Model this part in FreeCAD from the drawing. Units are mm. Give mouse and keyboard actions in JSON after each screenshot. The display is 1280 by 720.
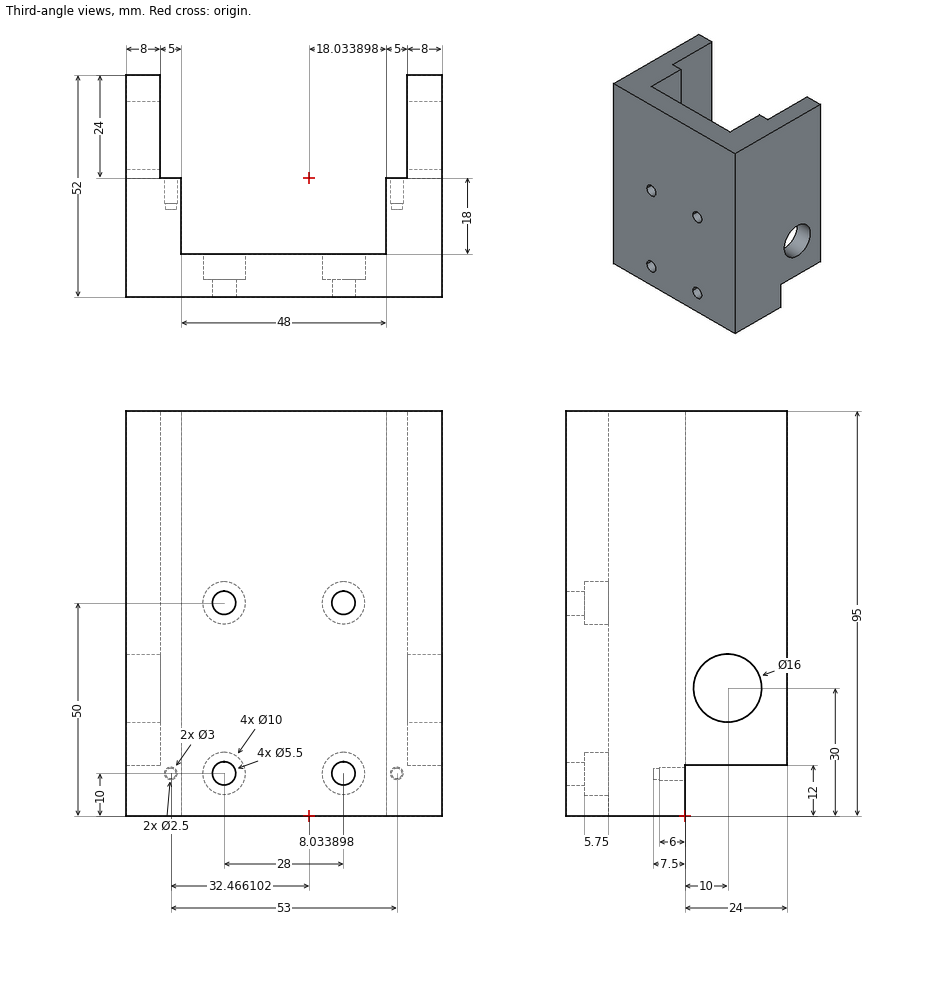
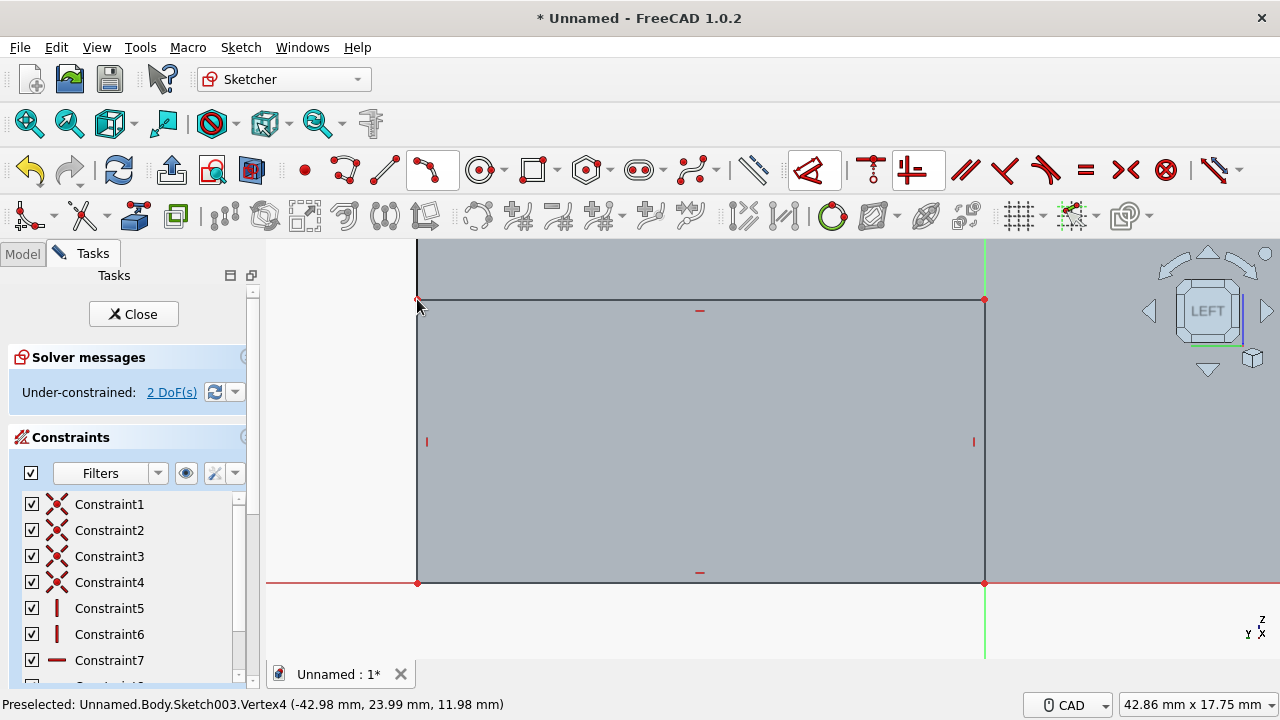
{"action": "left_click", "coordinate": [985, 498]}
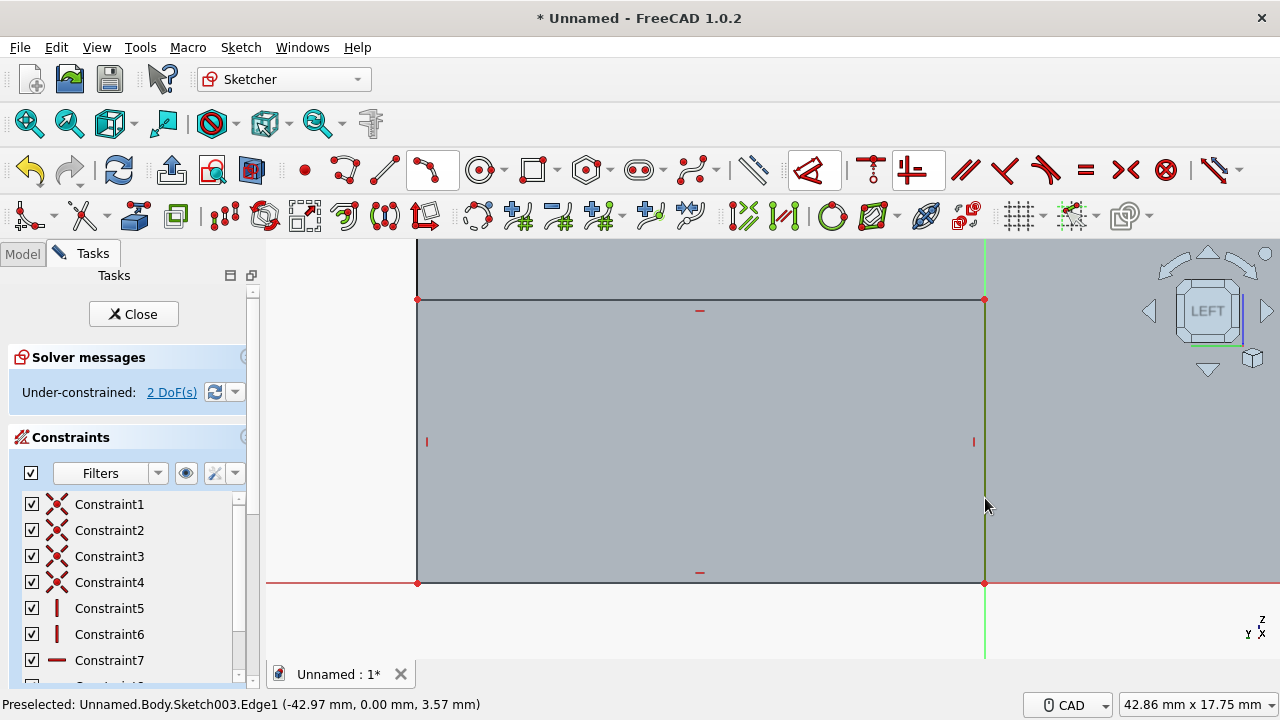
{"action": "key", "text": "i"}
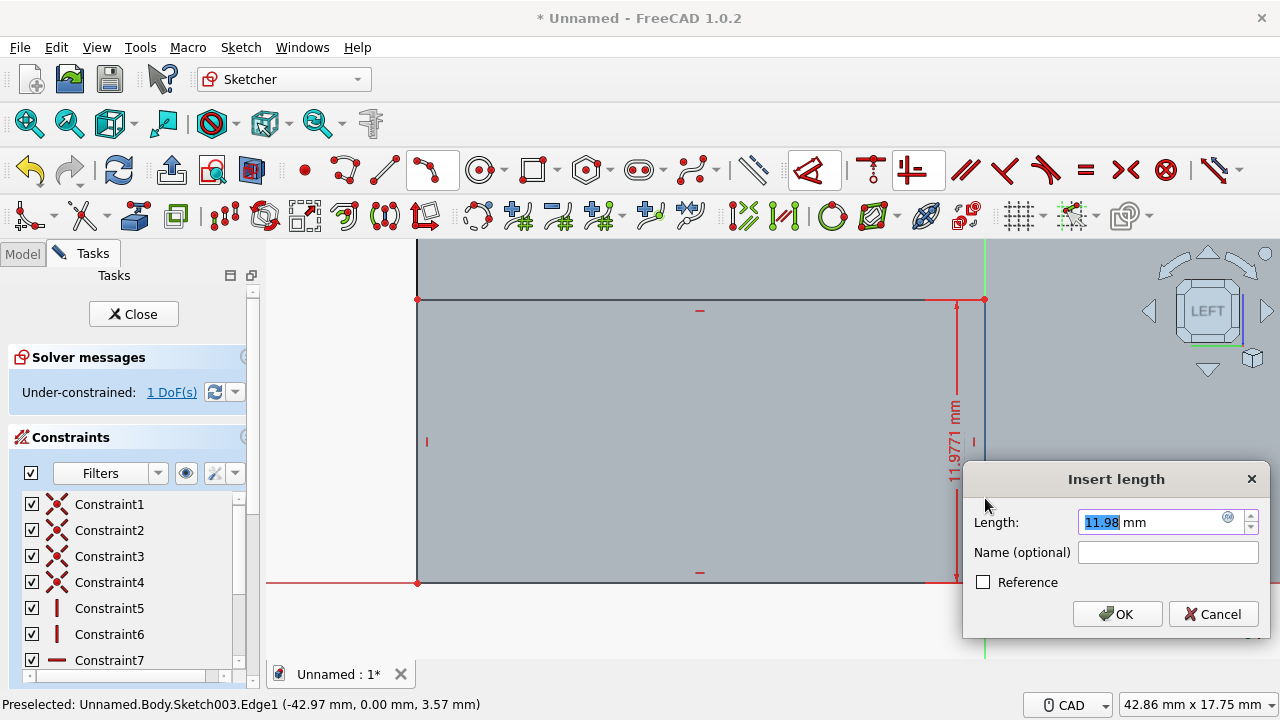
{"action": "type", "text": "12"}
{"action": "key", "text": "Return"}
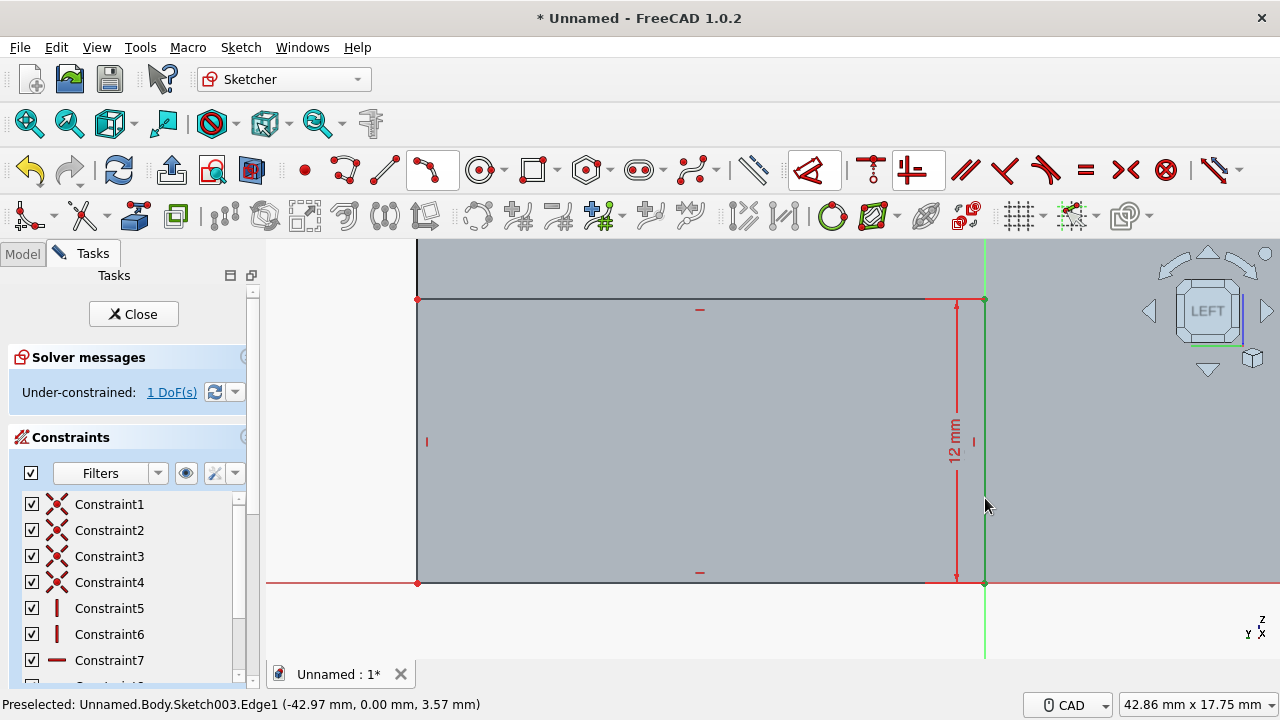
{"action": "left_click", "coordinate": [814, 299]}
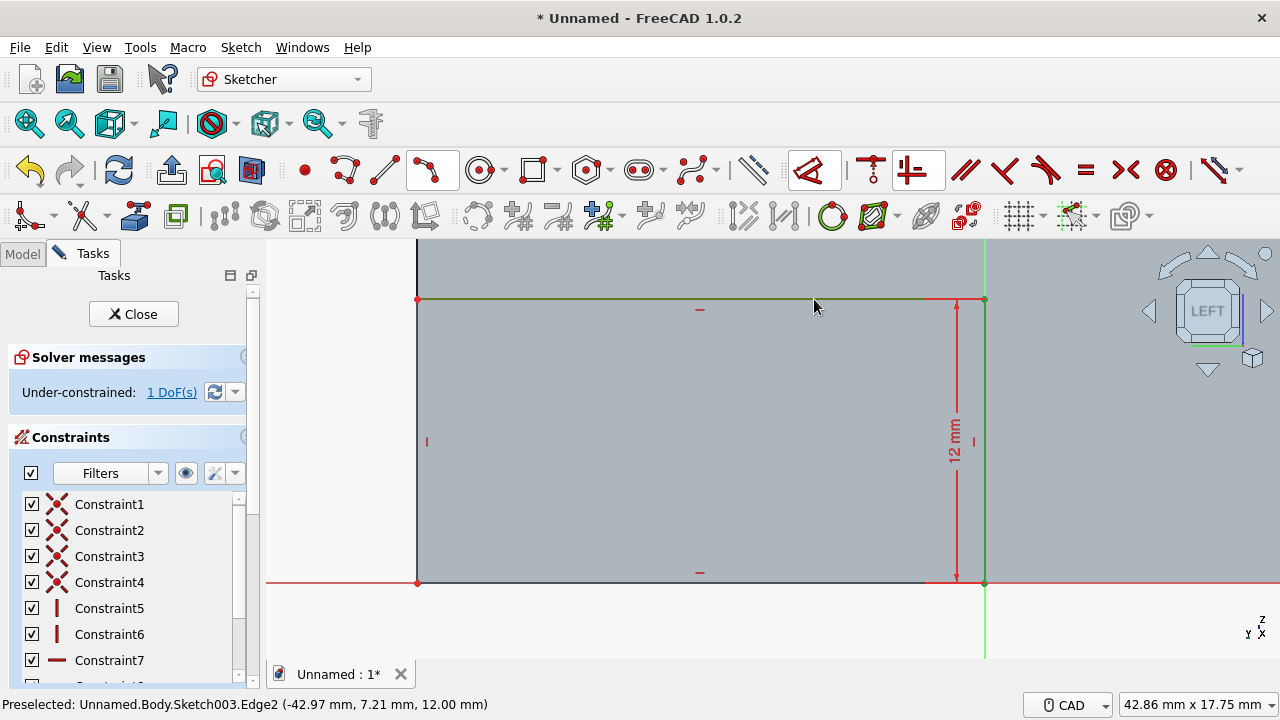
{"action": "left_click", "coordinate": [836, 170]}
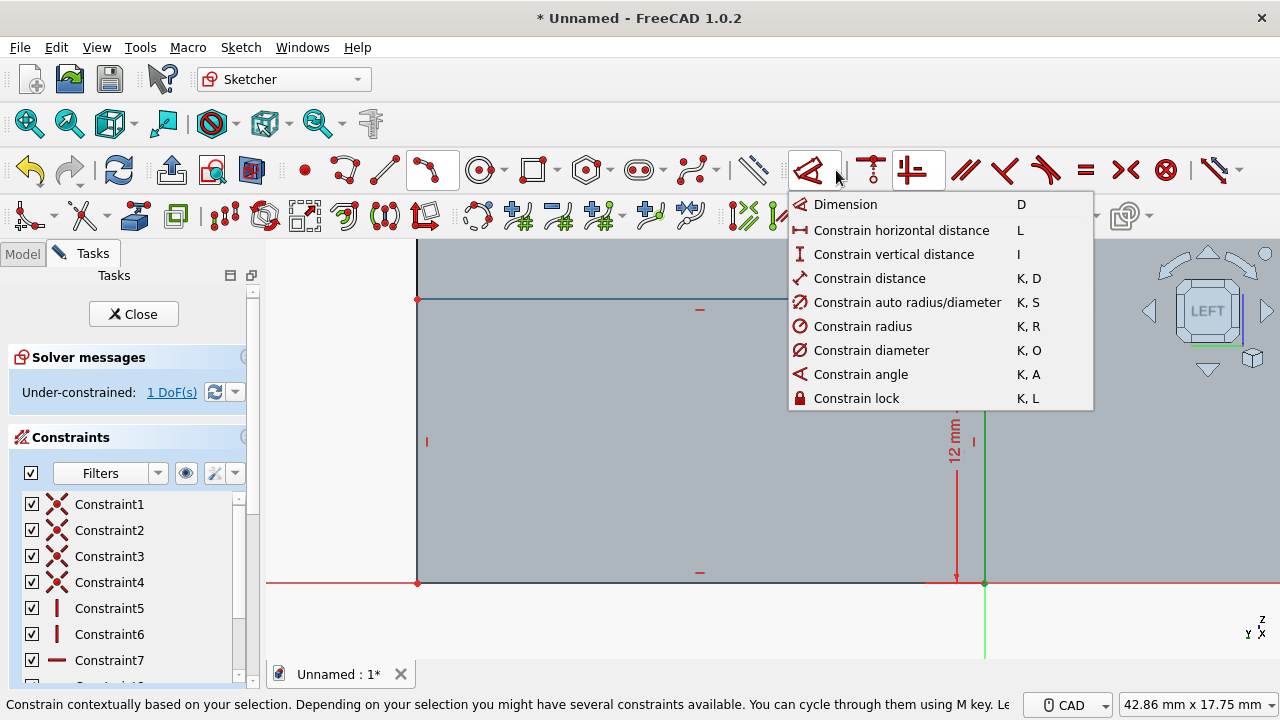
{"action": "left_click", "coordinate": [941, 230]}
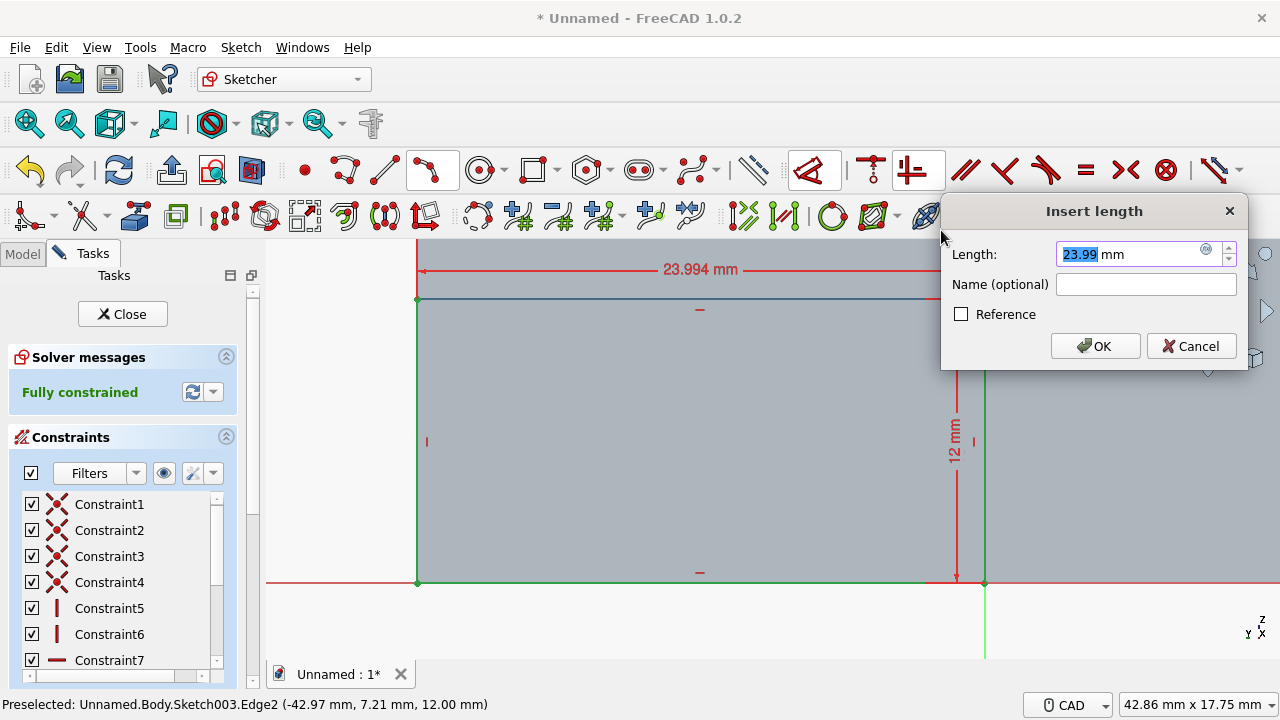
{"action": "type", "text": "24"}
{"action": "key", "text": "Return"}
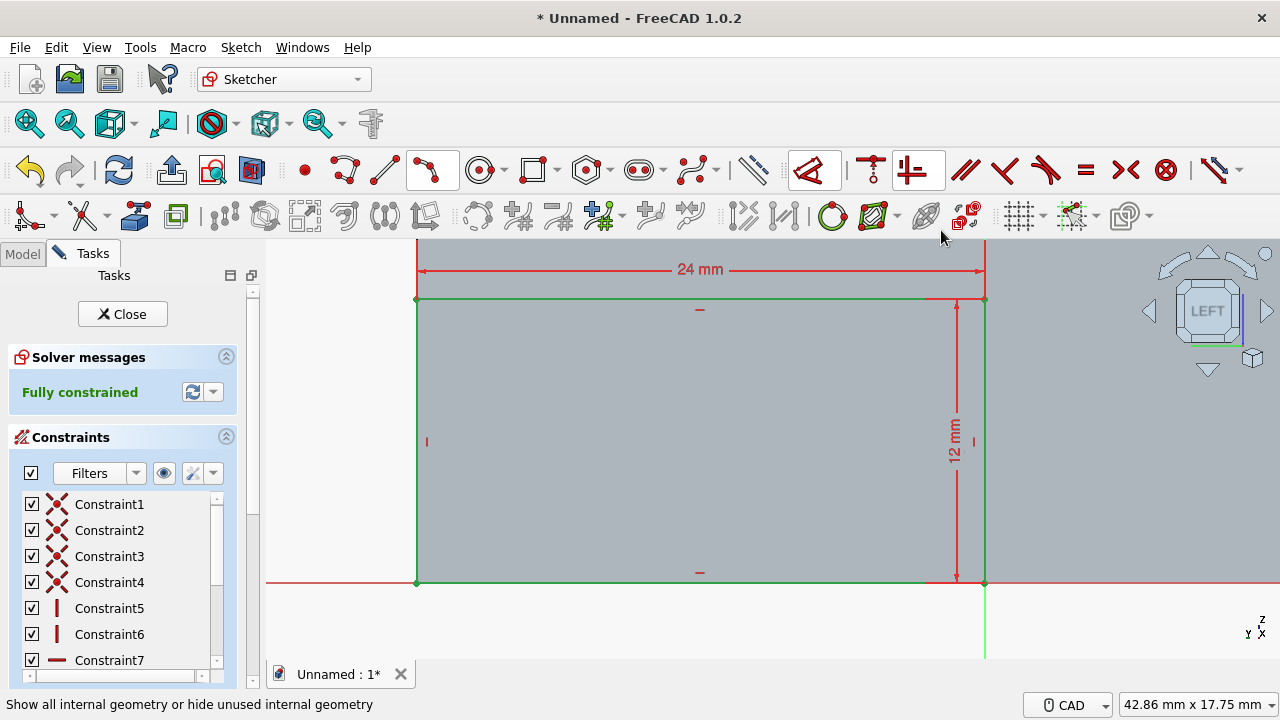
{"action": "left_click", "coordinate": [123, 314]}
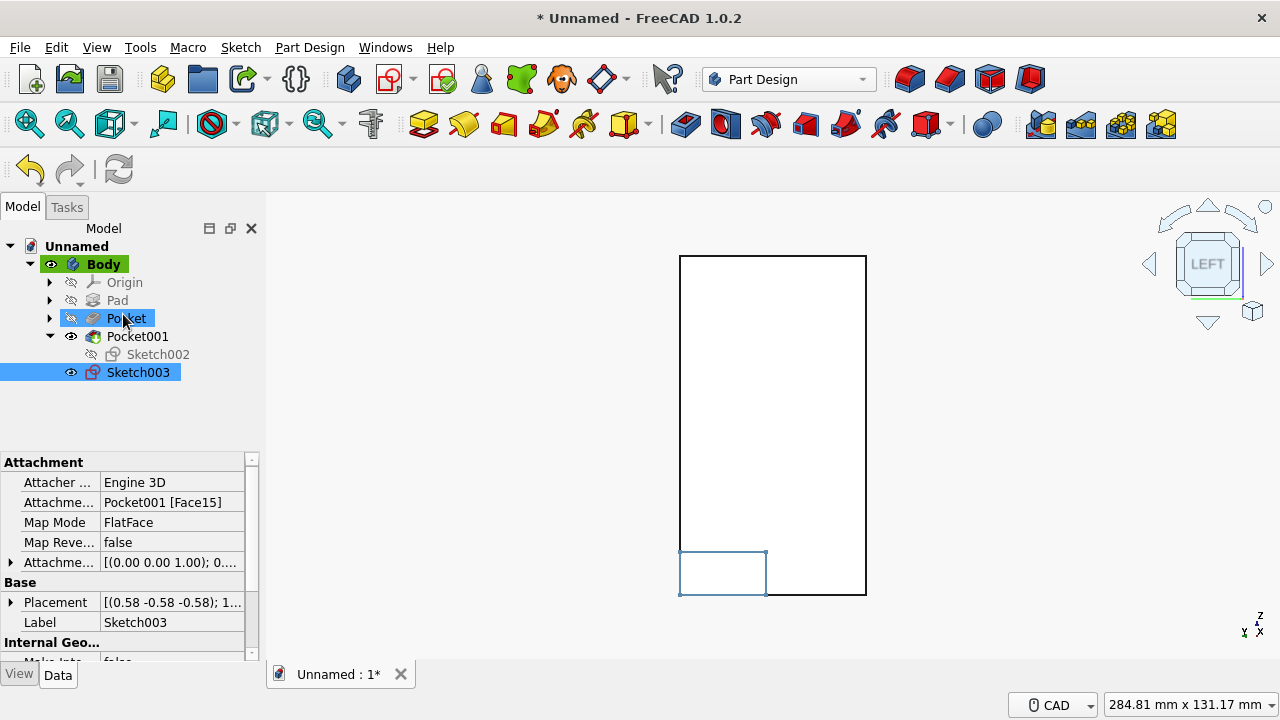
{"action": "left_click", "coordinate": [686, 124]}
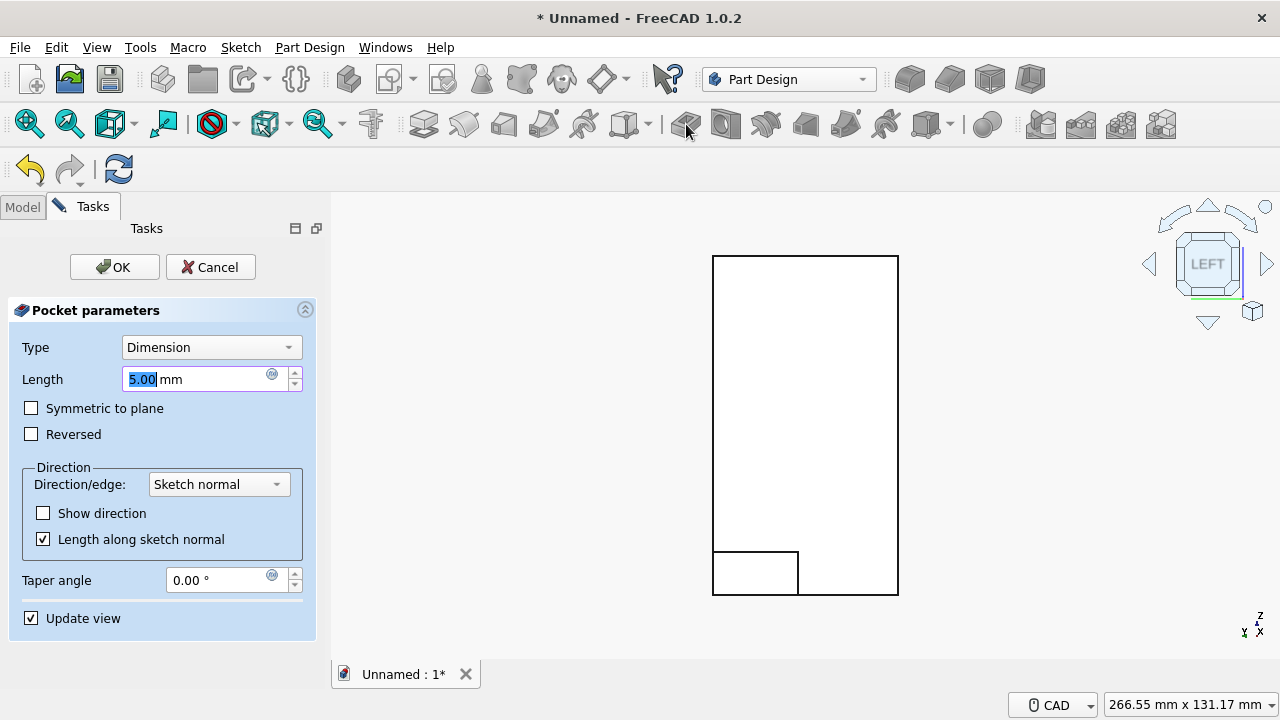
{"action": "left_click", "coordinate": [212, 348]}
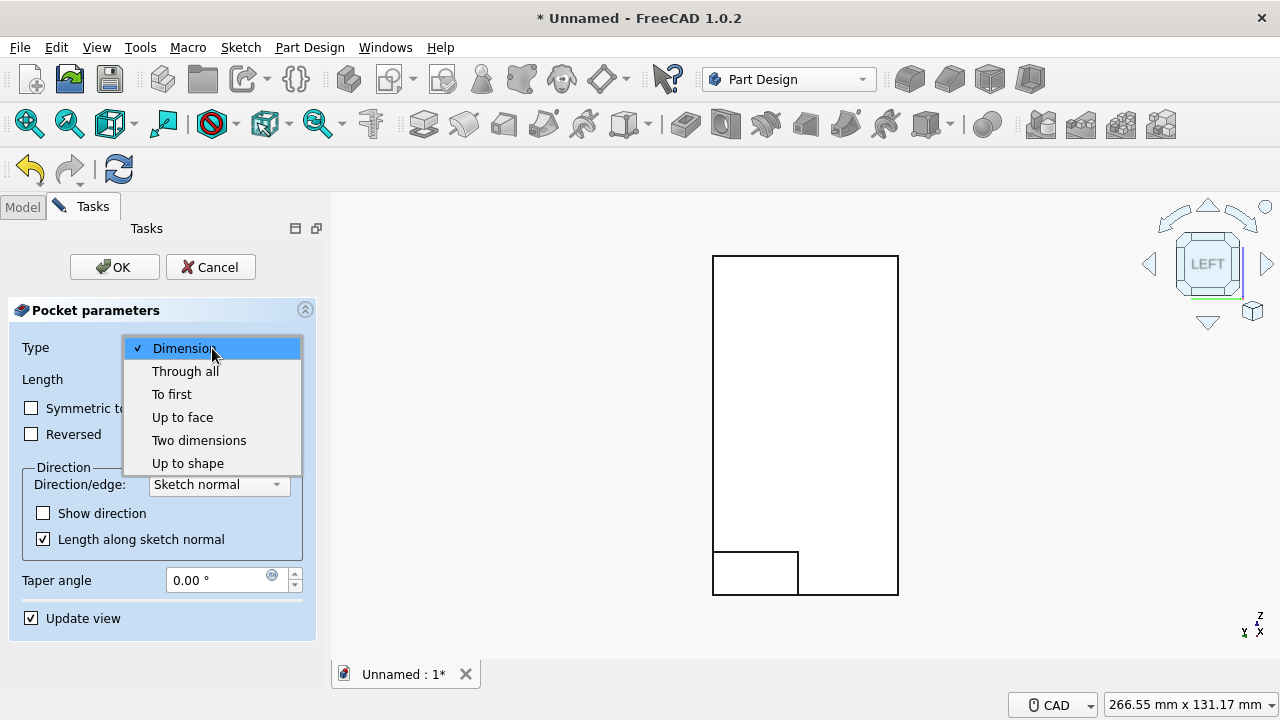
{"action": "left_click", "coordinate": [212, 372]}